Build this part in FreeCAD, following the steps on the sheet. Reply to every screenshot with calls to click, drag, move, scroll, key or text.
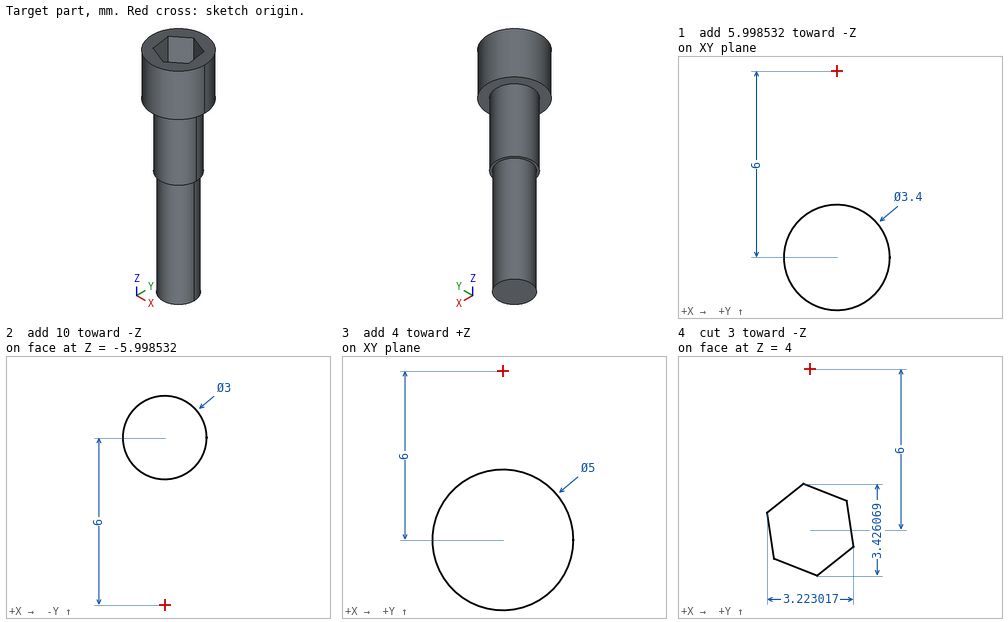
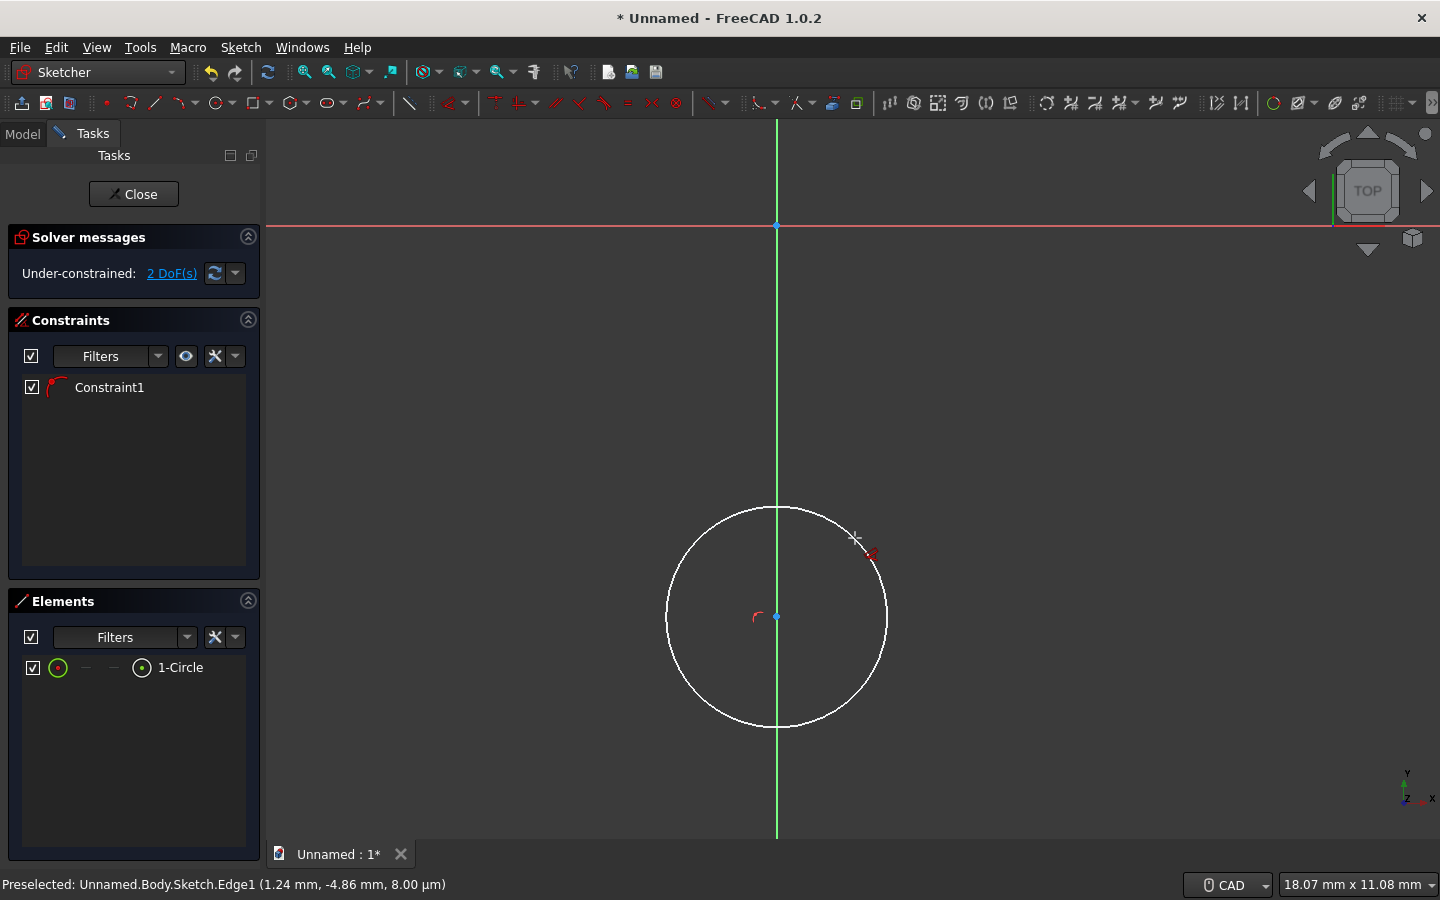
click(855, 539)
click(878, 516)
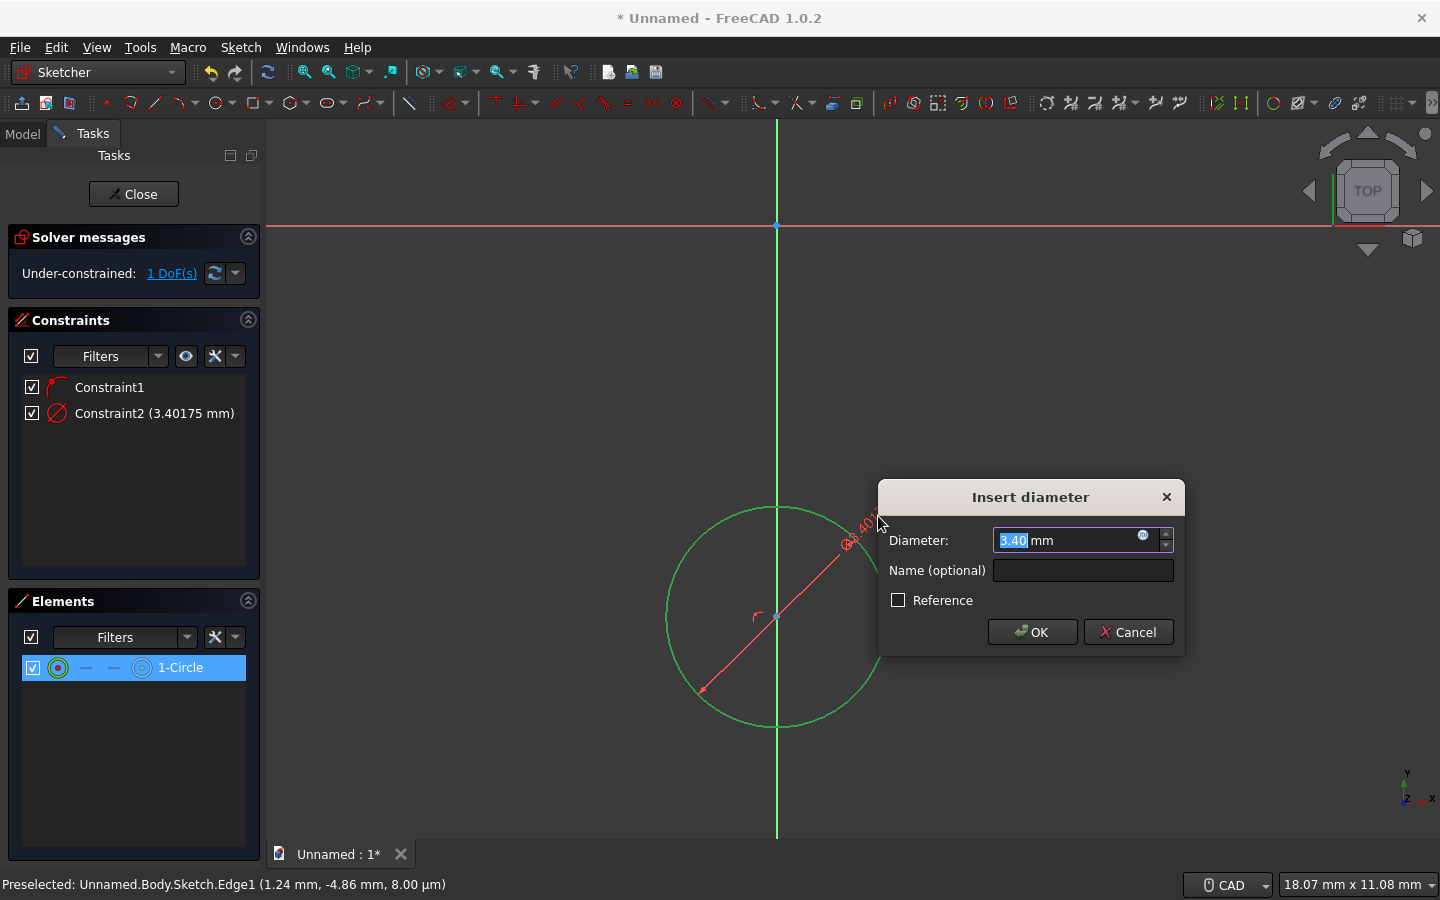
text(3.4)
key(Return)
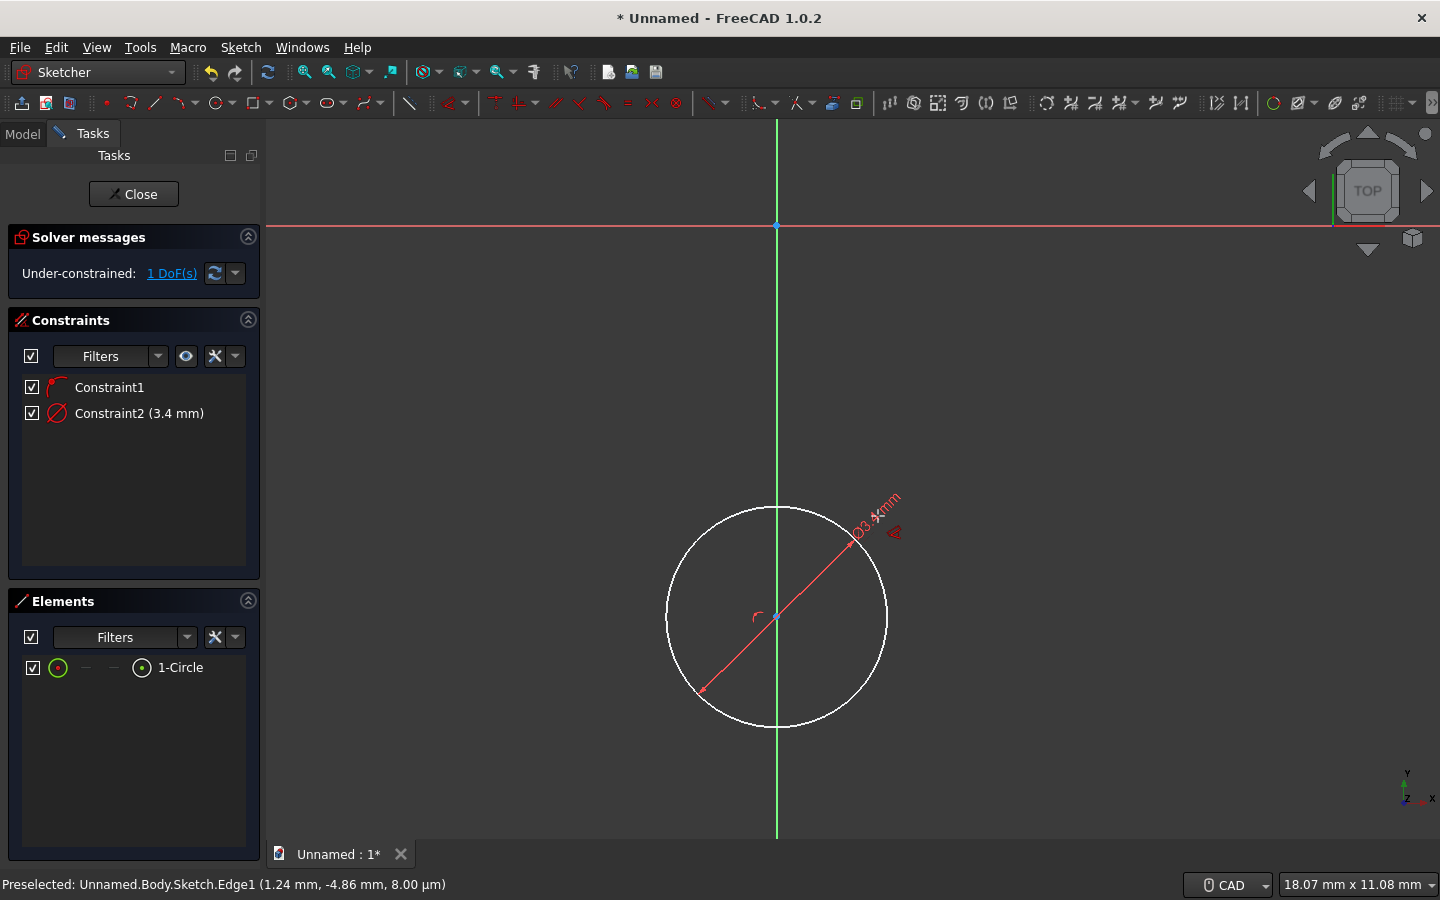
click(777, 617)
click(811, 421)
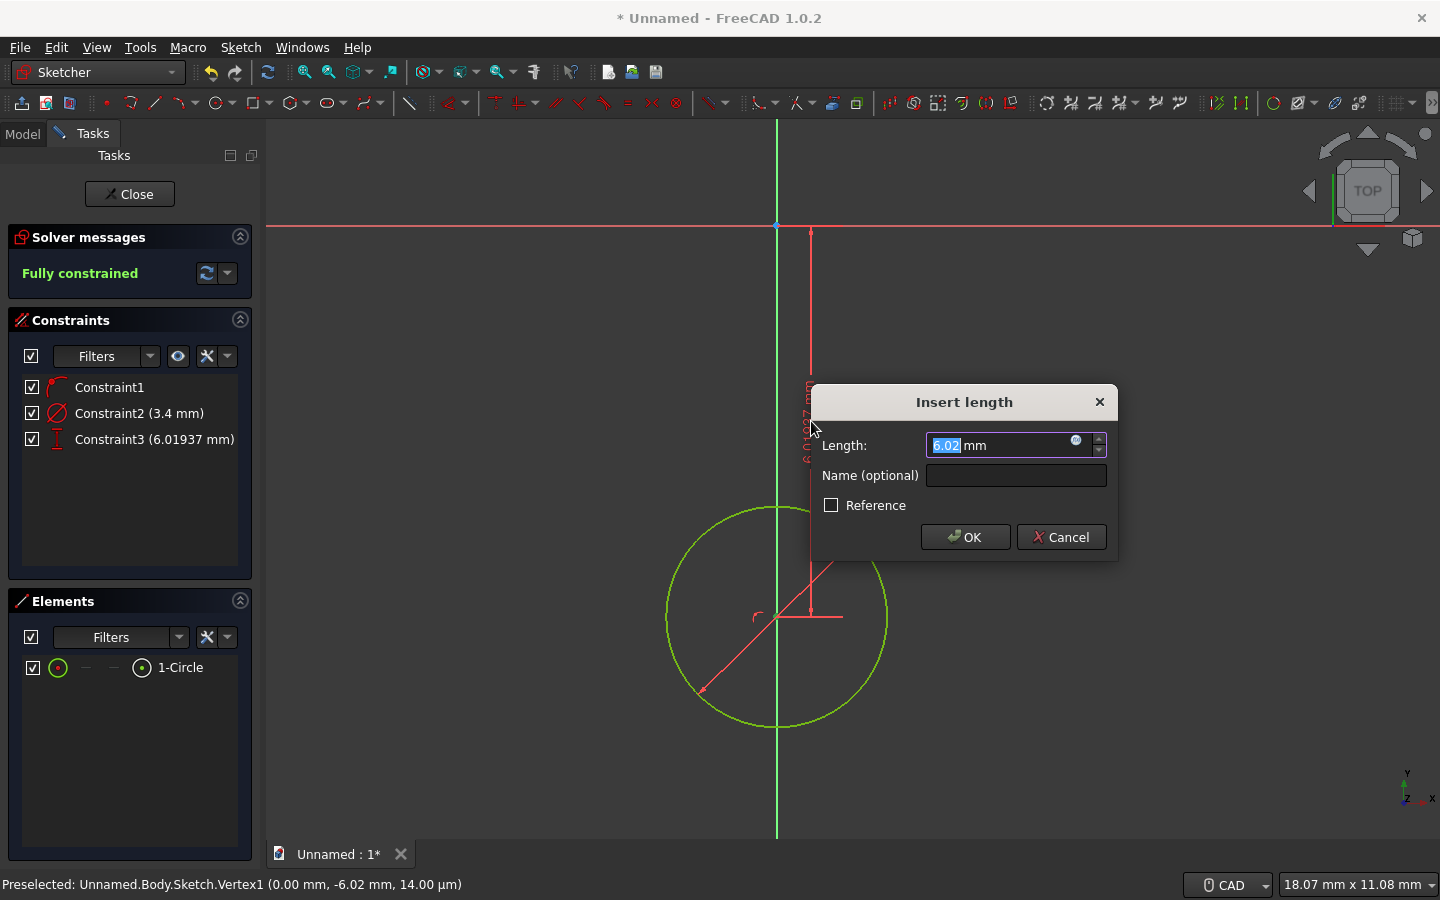
text(6)
key(Return)
key(Escape)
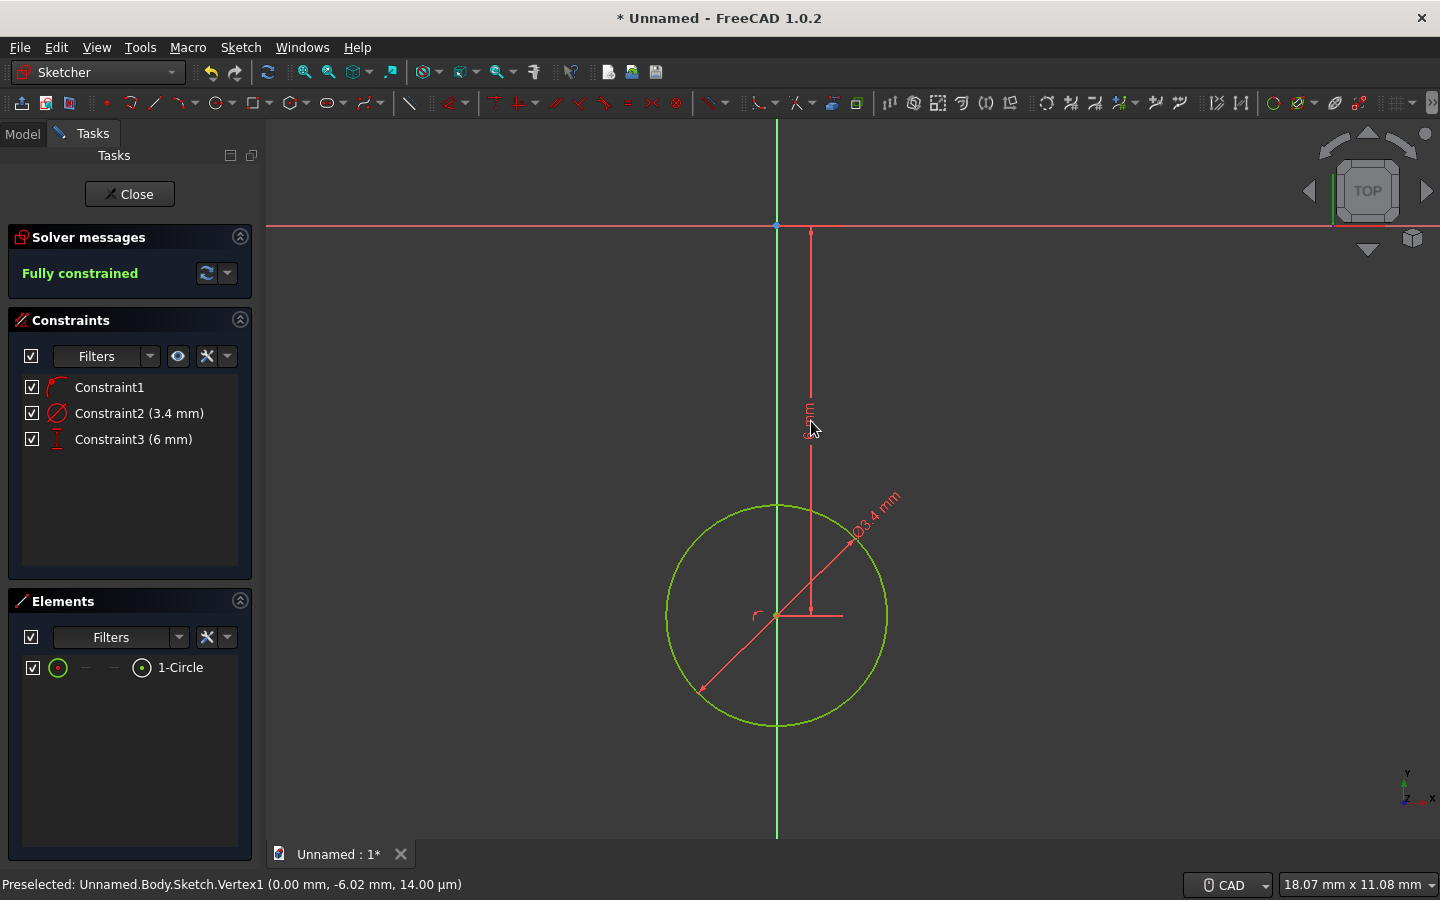
click(130, 194)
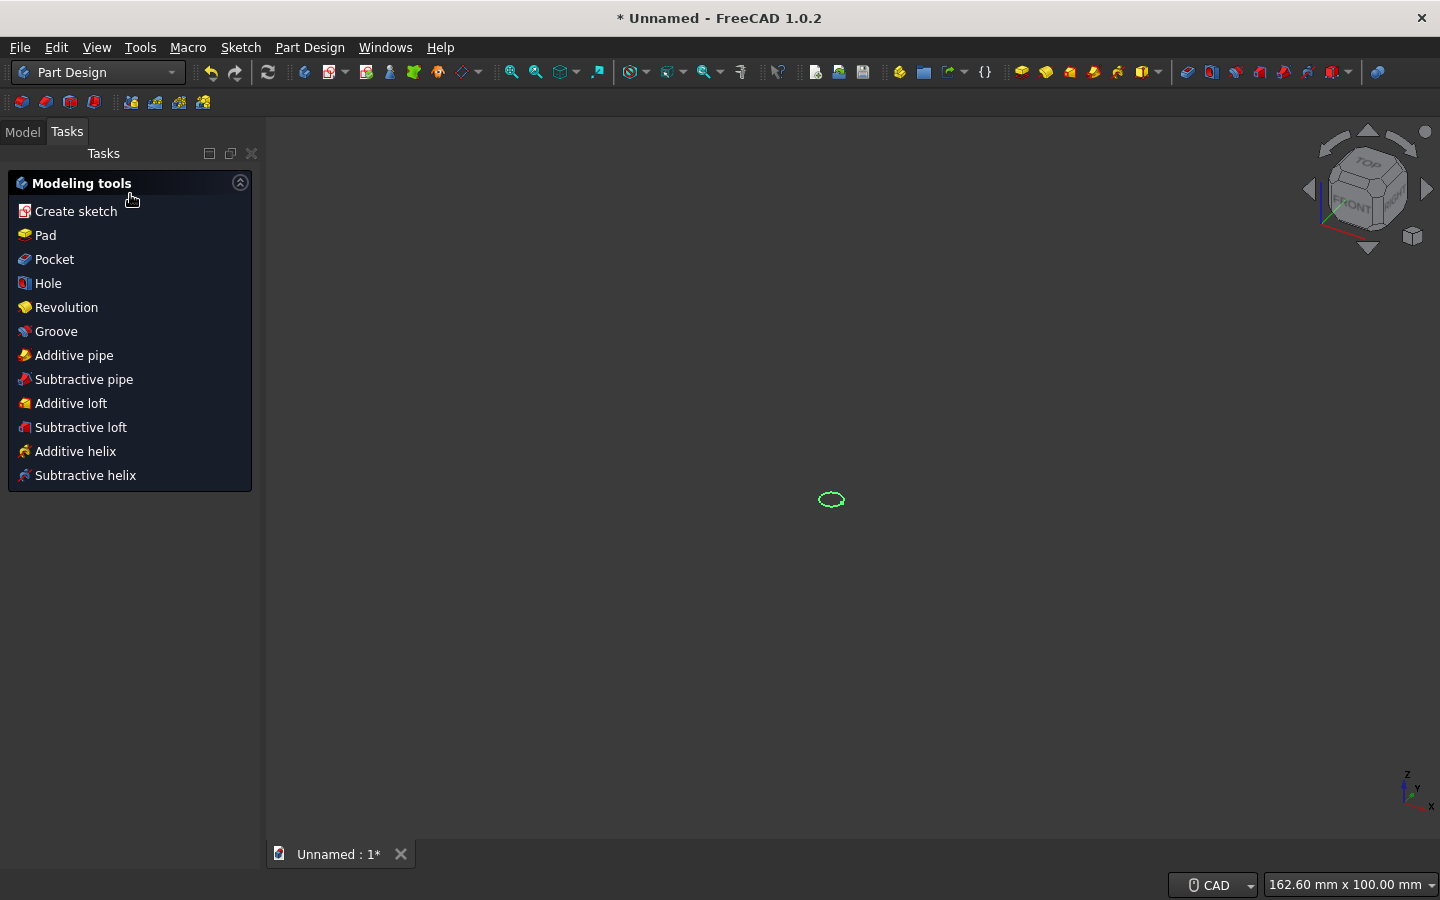
click(1022, 72)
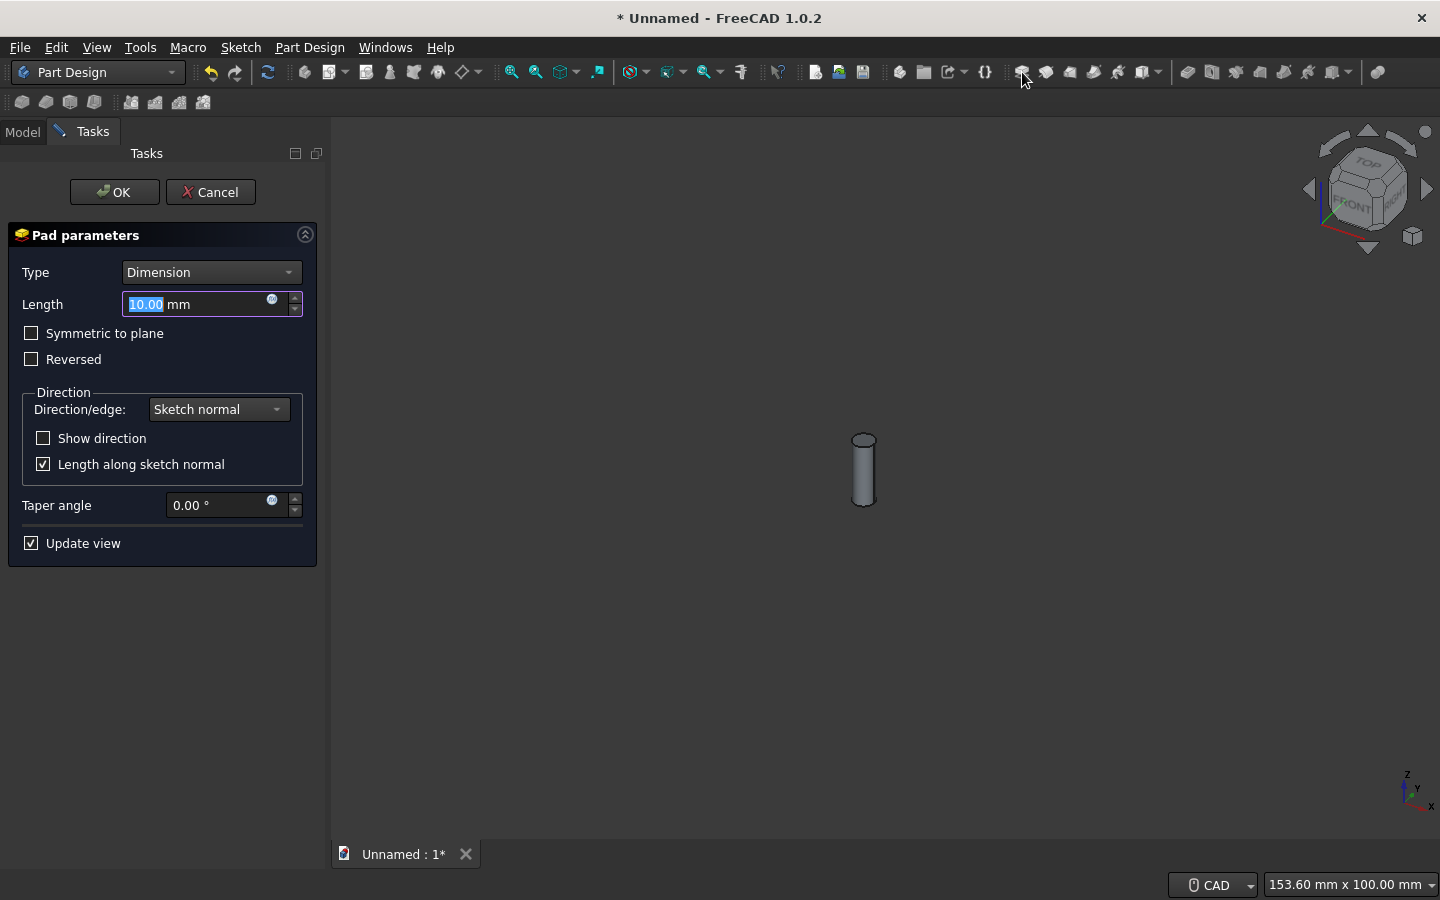
text(5.998532)
key(Tab)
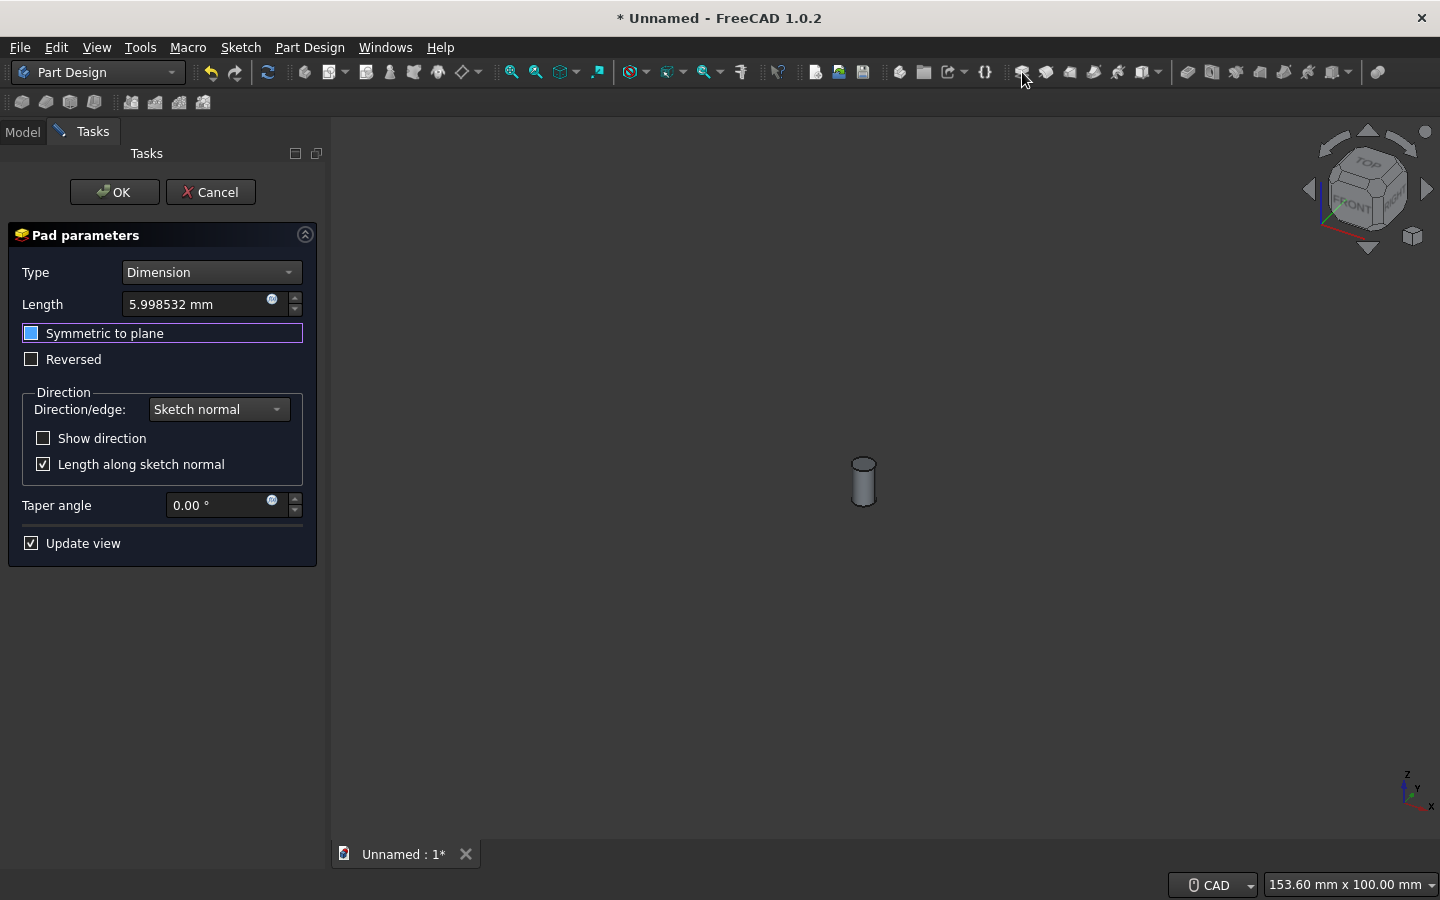
click(30, 359)